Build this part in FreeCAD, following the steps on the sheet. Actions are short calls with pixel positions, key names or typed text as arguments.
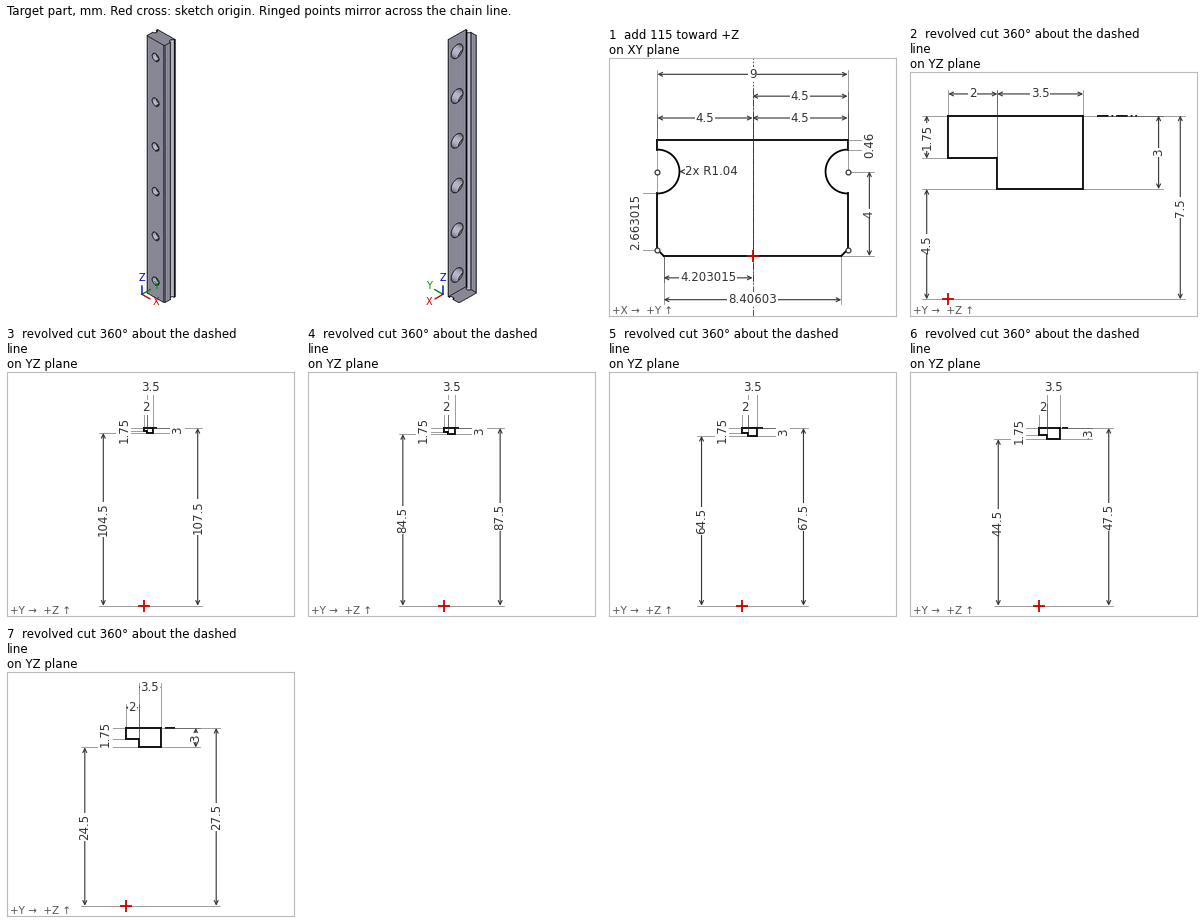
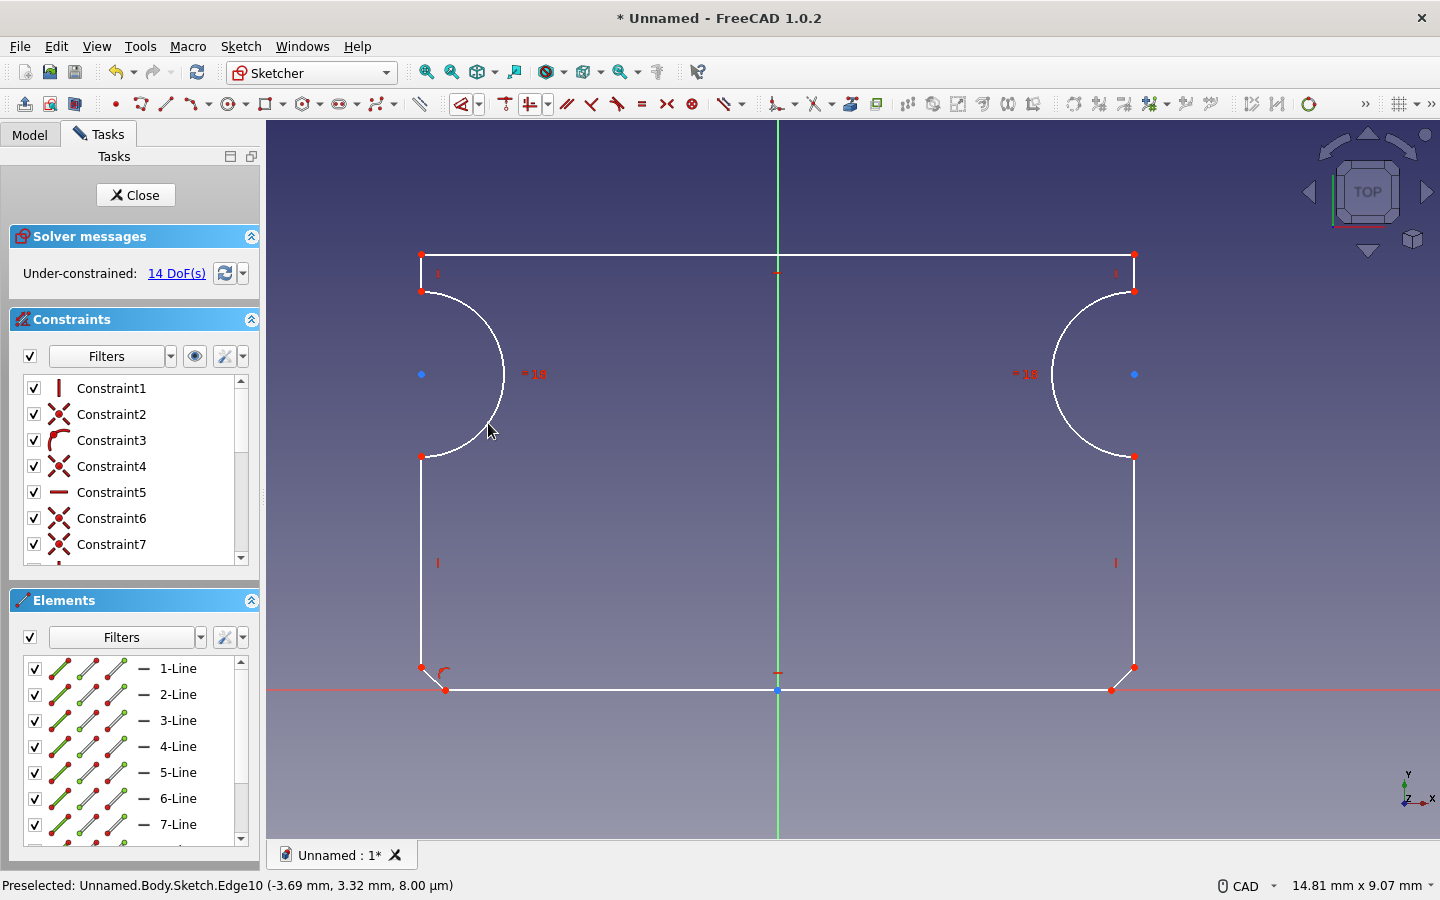
click(1135, 375)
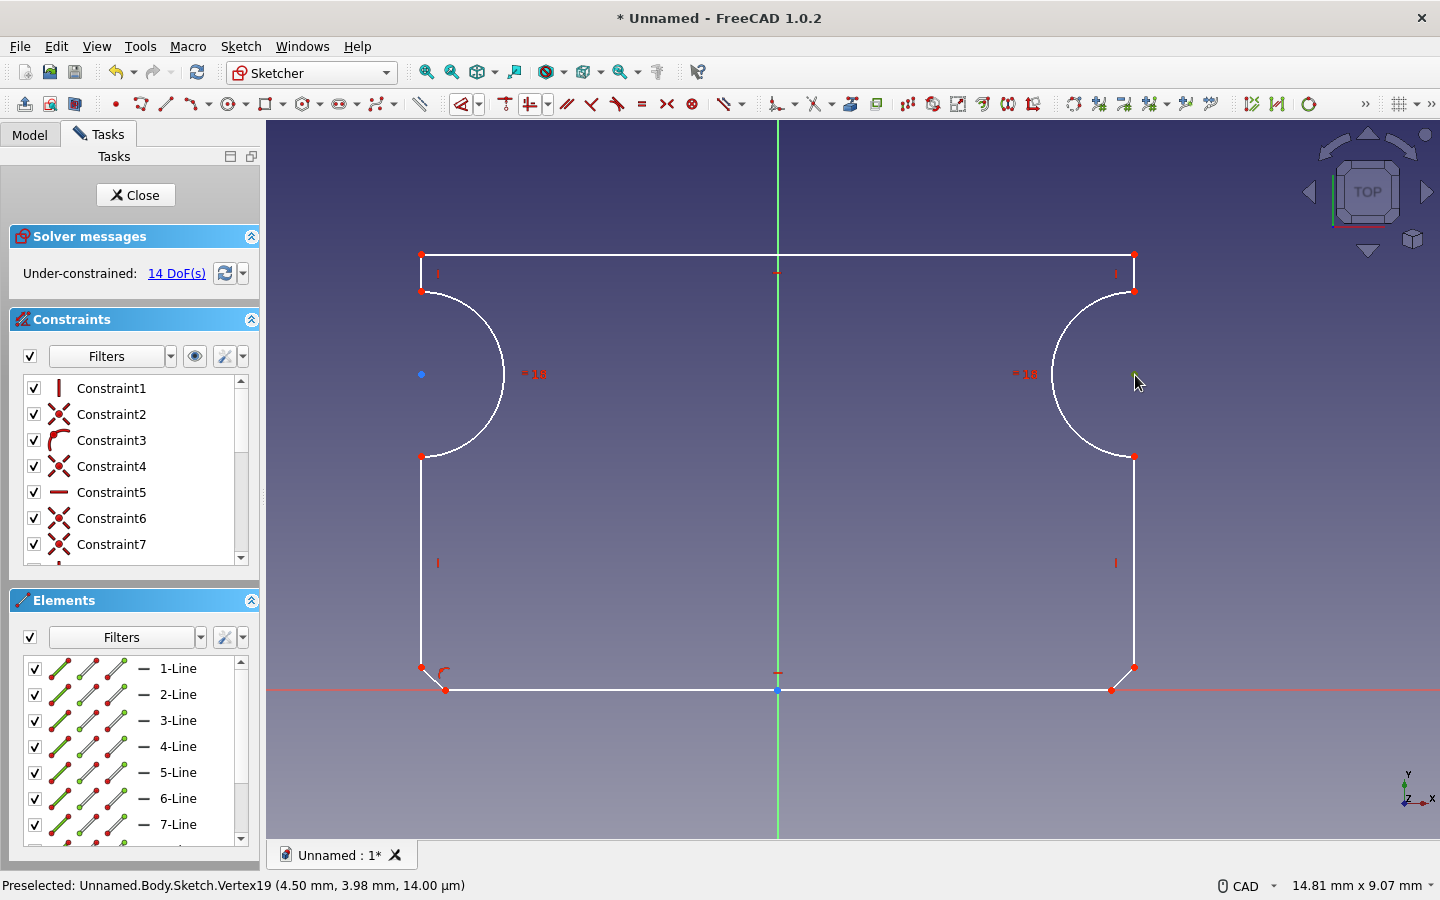
click(422, 375)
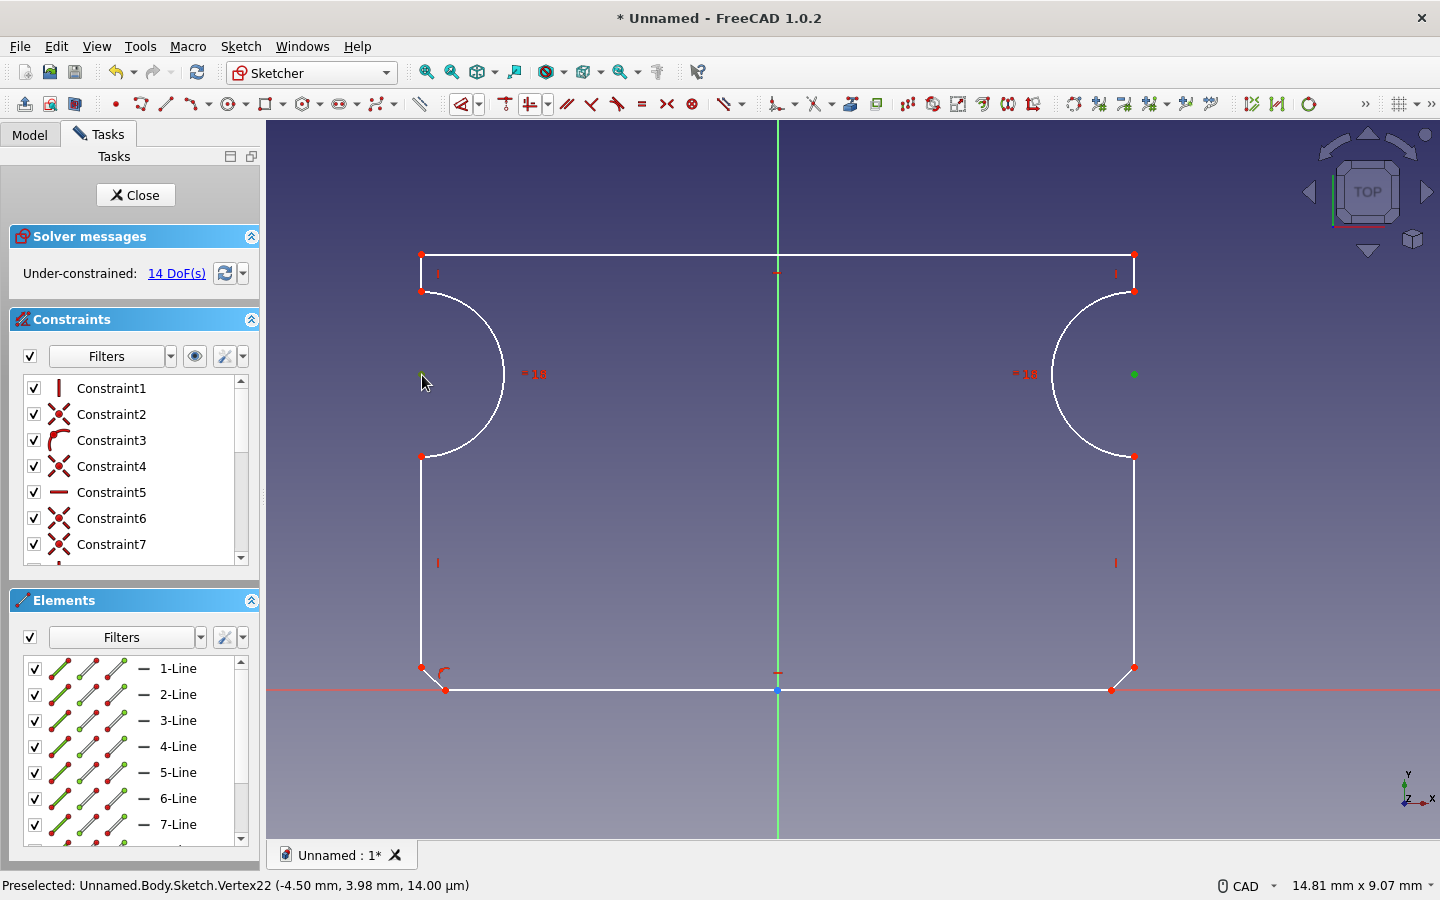
click(778, 764)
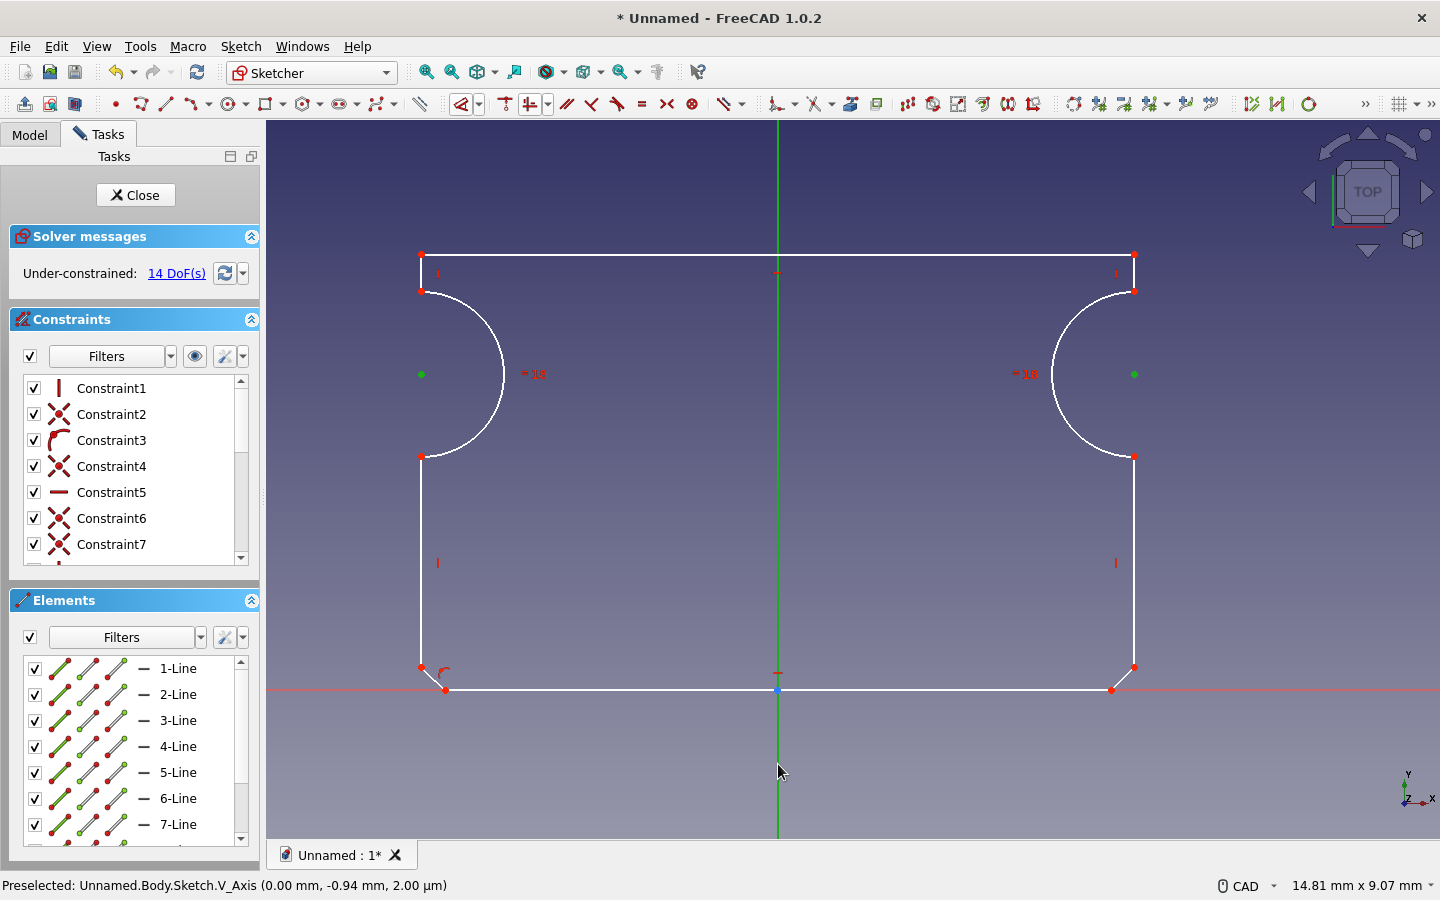
key(s)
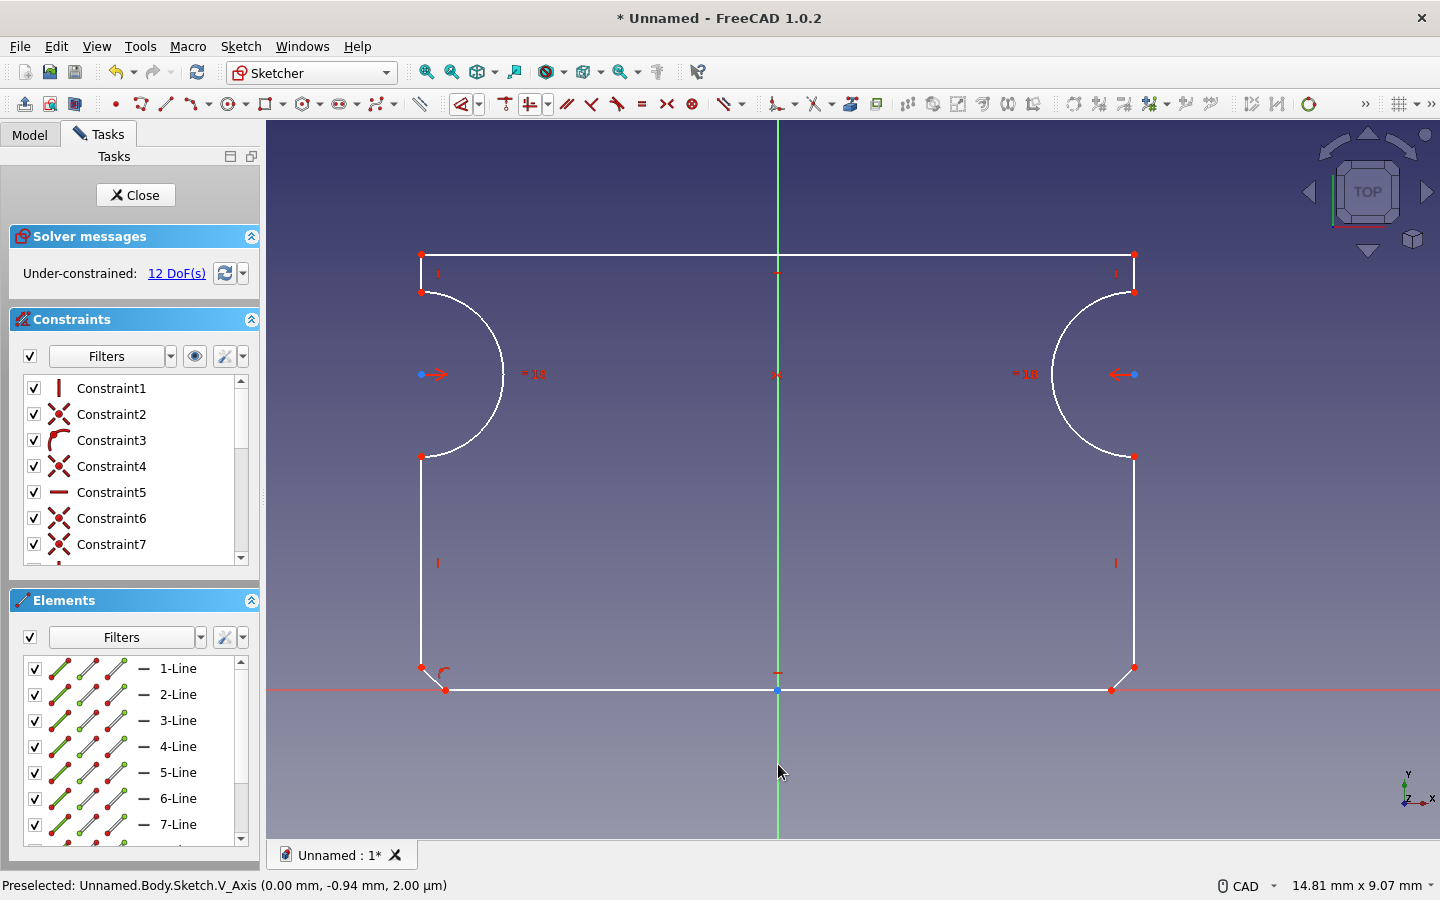
click(421, 668)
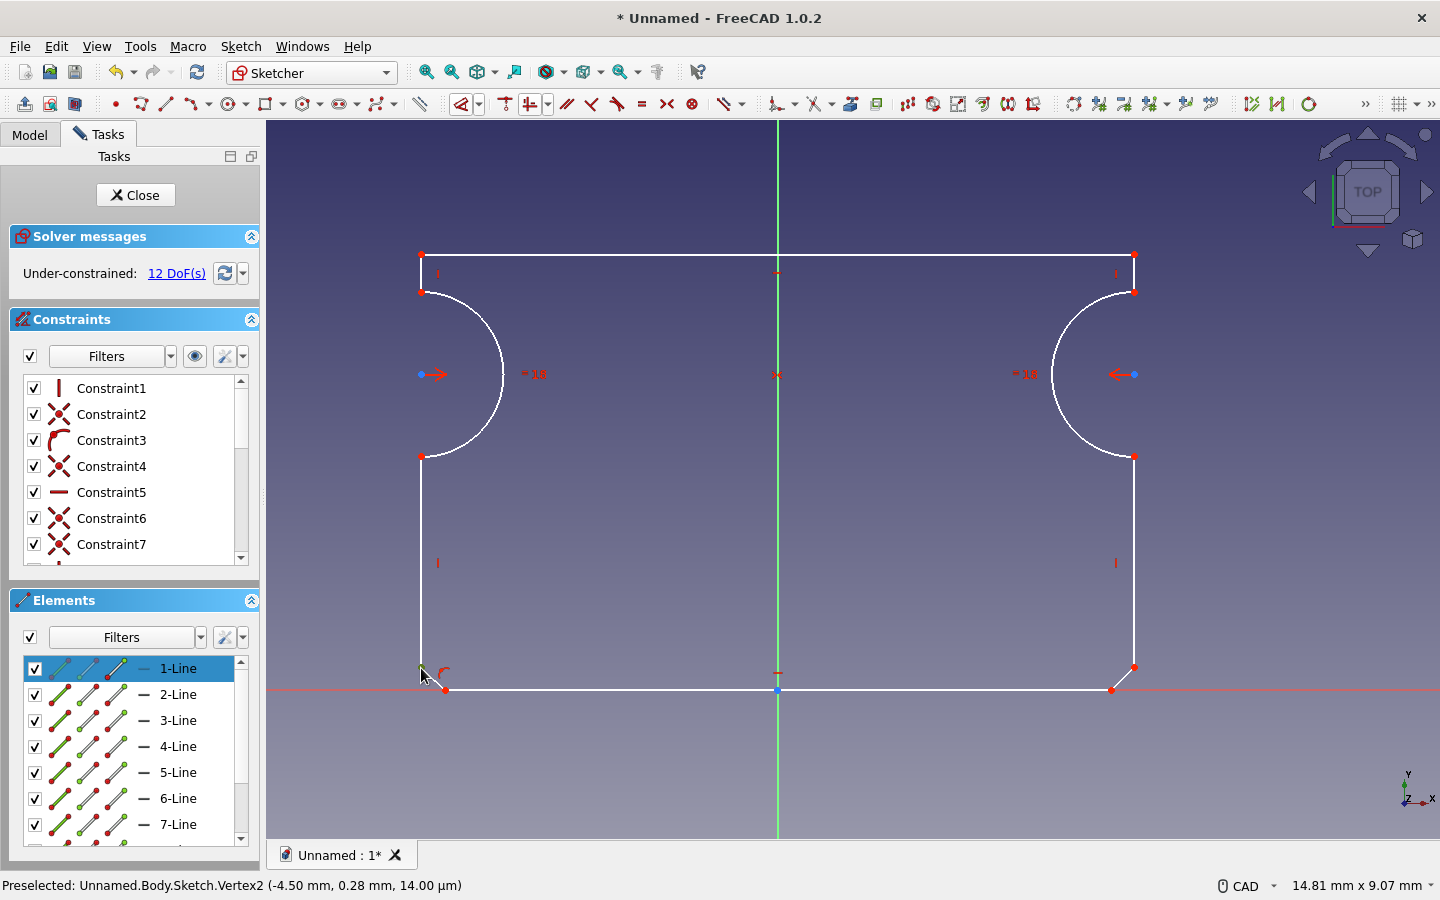
click(1134, 668)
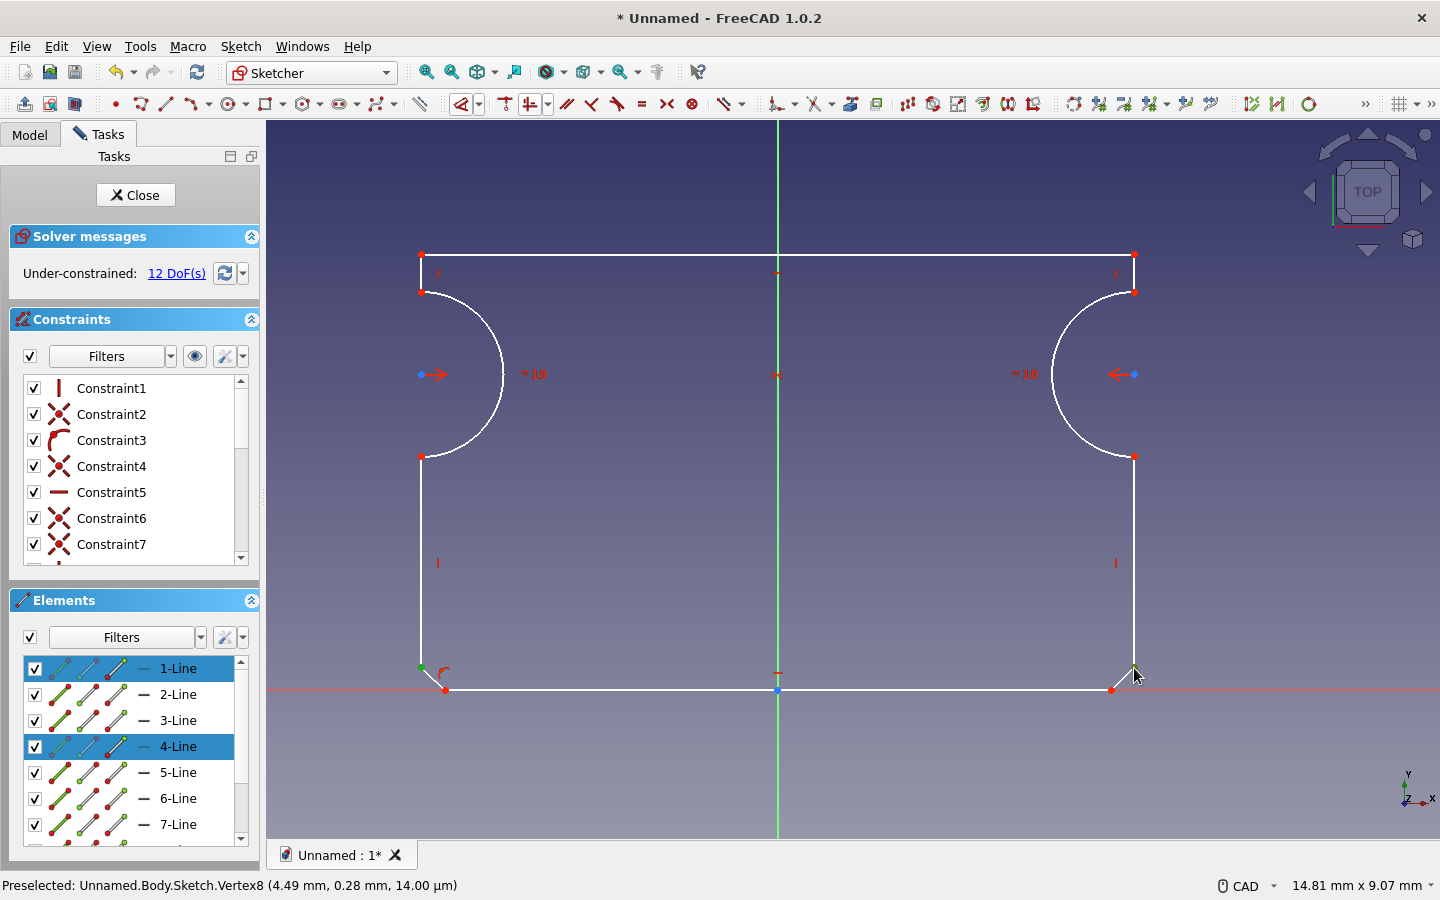
click(778, 764)